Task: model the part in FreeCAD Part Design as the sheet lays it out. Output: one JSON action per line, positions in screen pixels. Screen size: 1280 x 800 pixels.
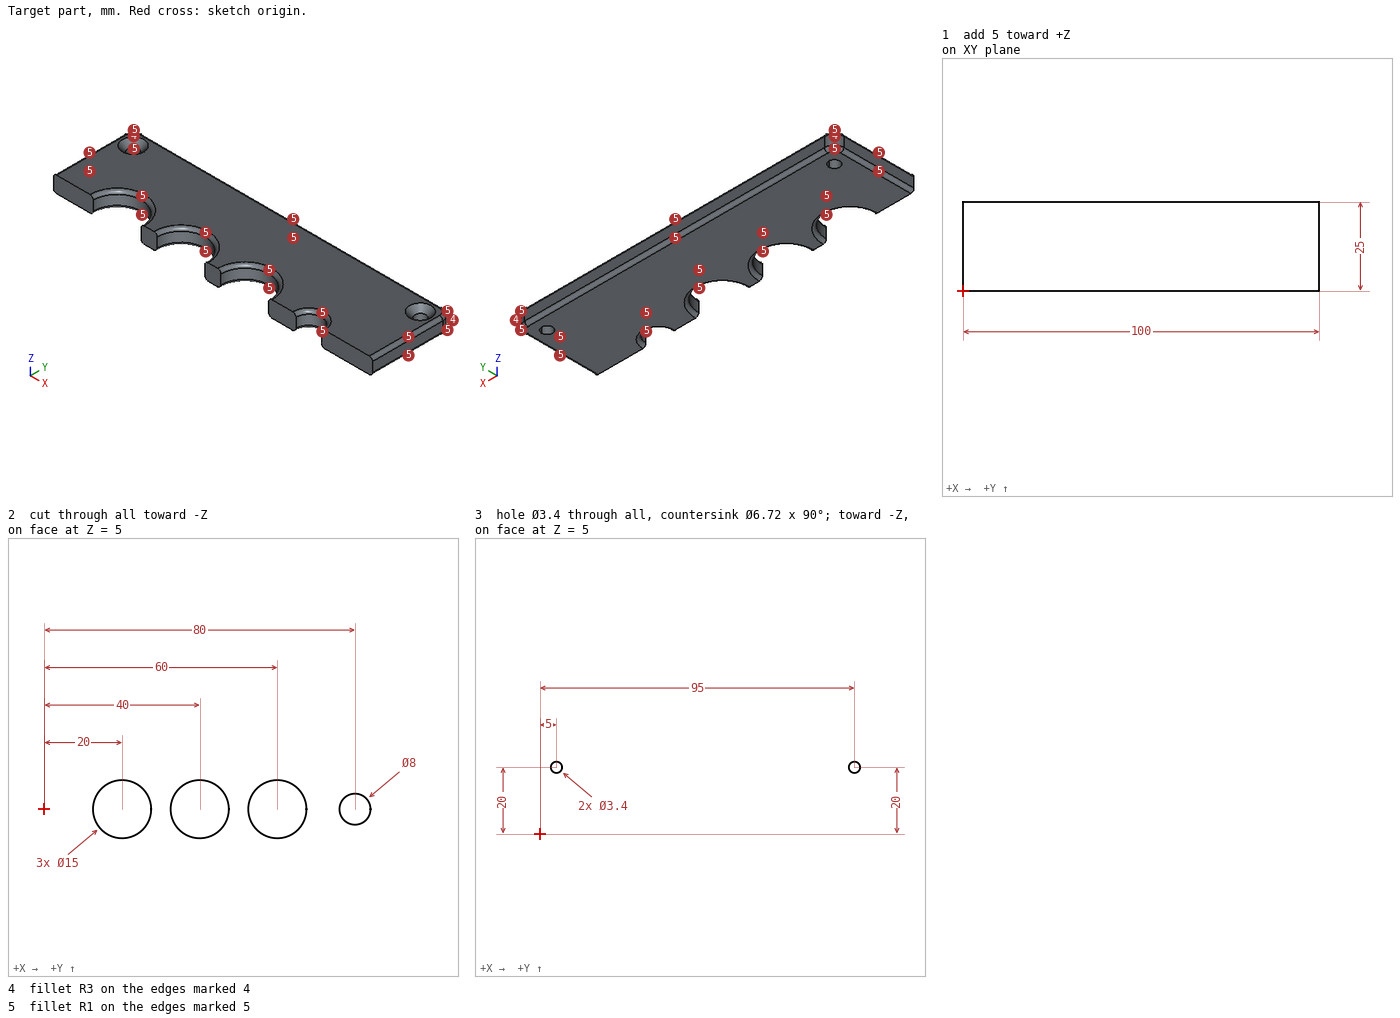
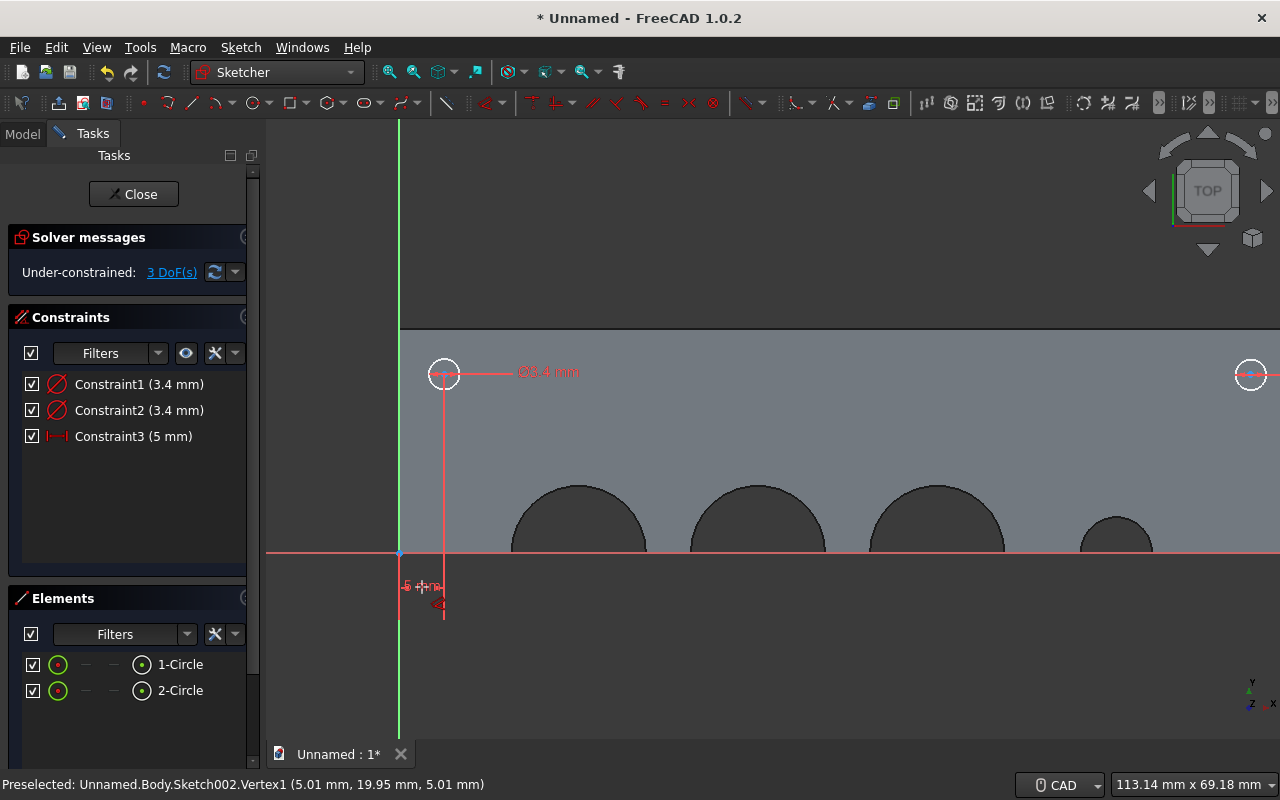
{"action": "left_click", "coordinate": [444, 374]}
{"action": "left_click", "coordinate": [365, 464]}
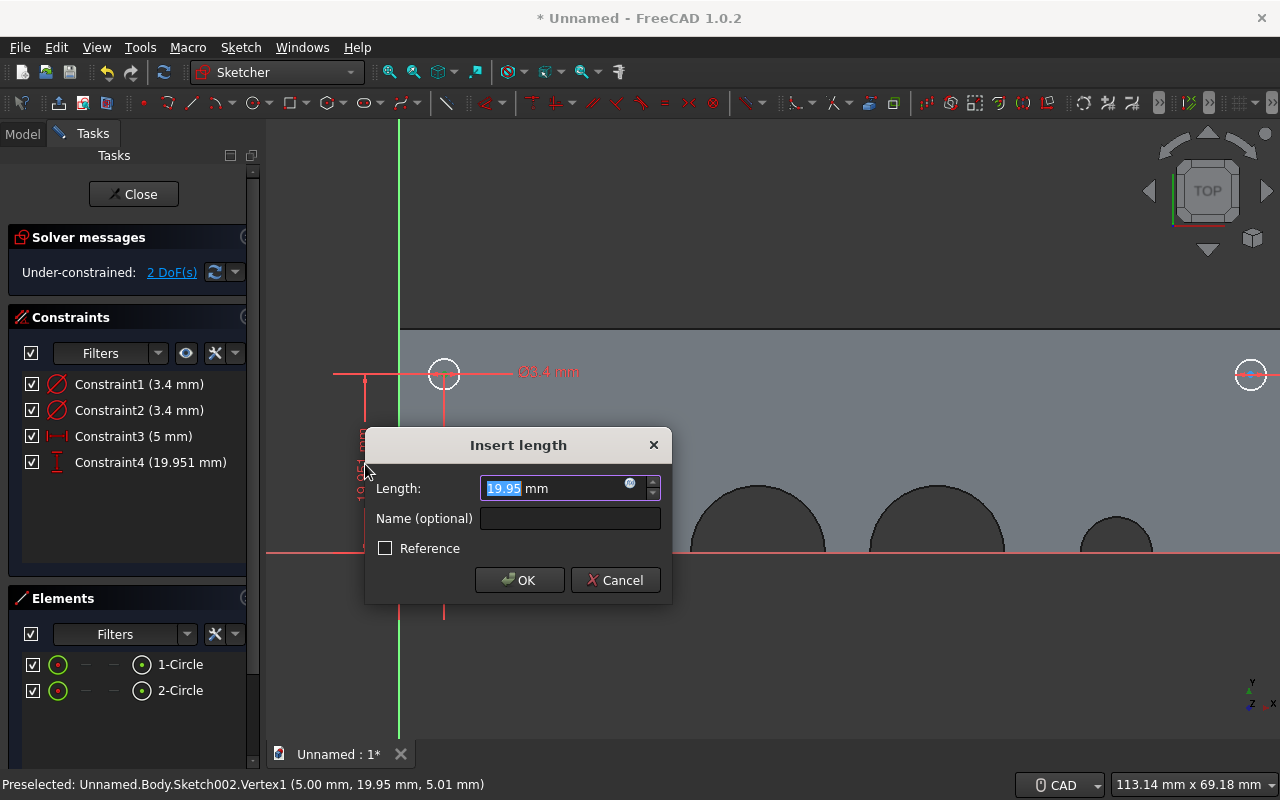
{"action": "type", "text": "20"}
{"action": "key", "text": "Return"}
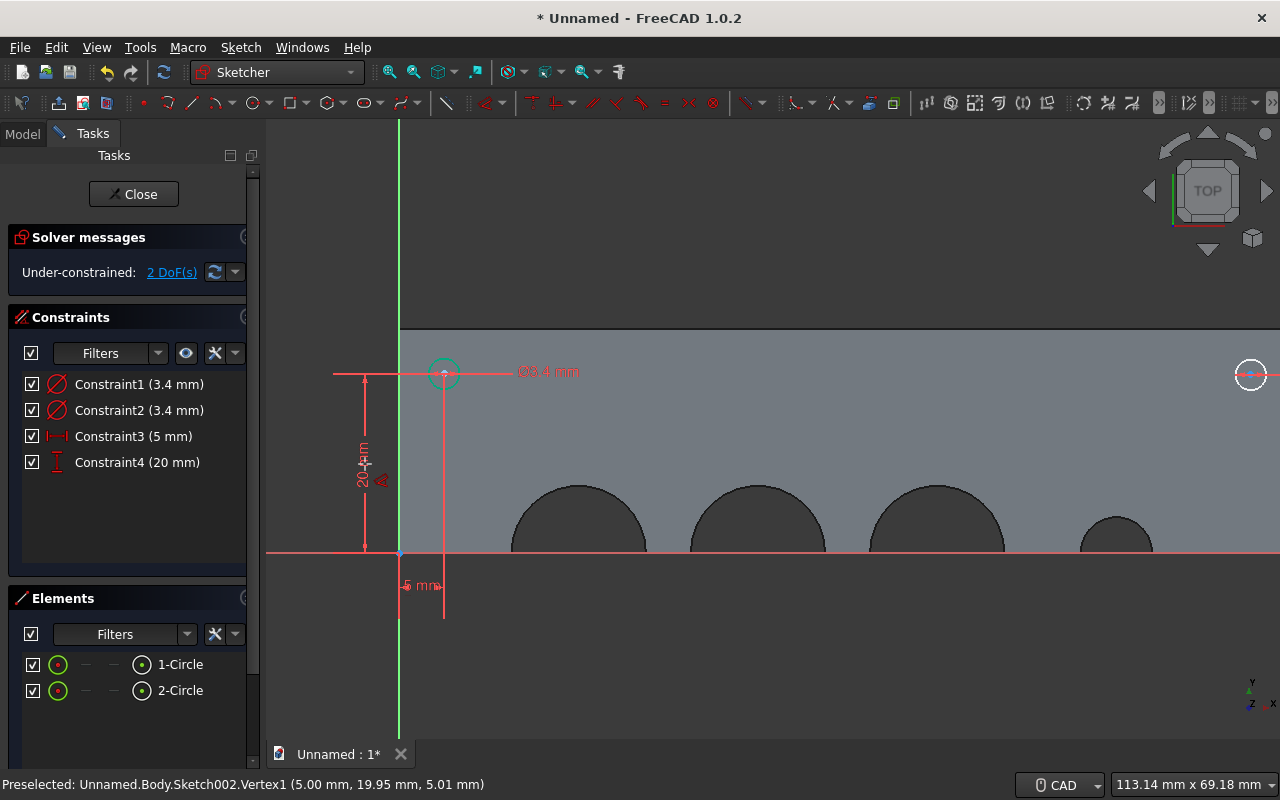
{"action": "scroll", "coordinate": [444, 374], "scroll_direction": "down", "scroll_amount": 2}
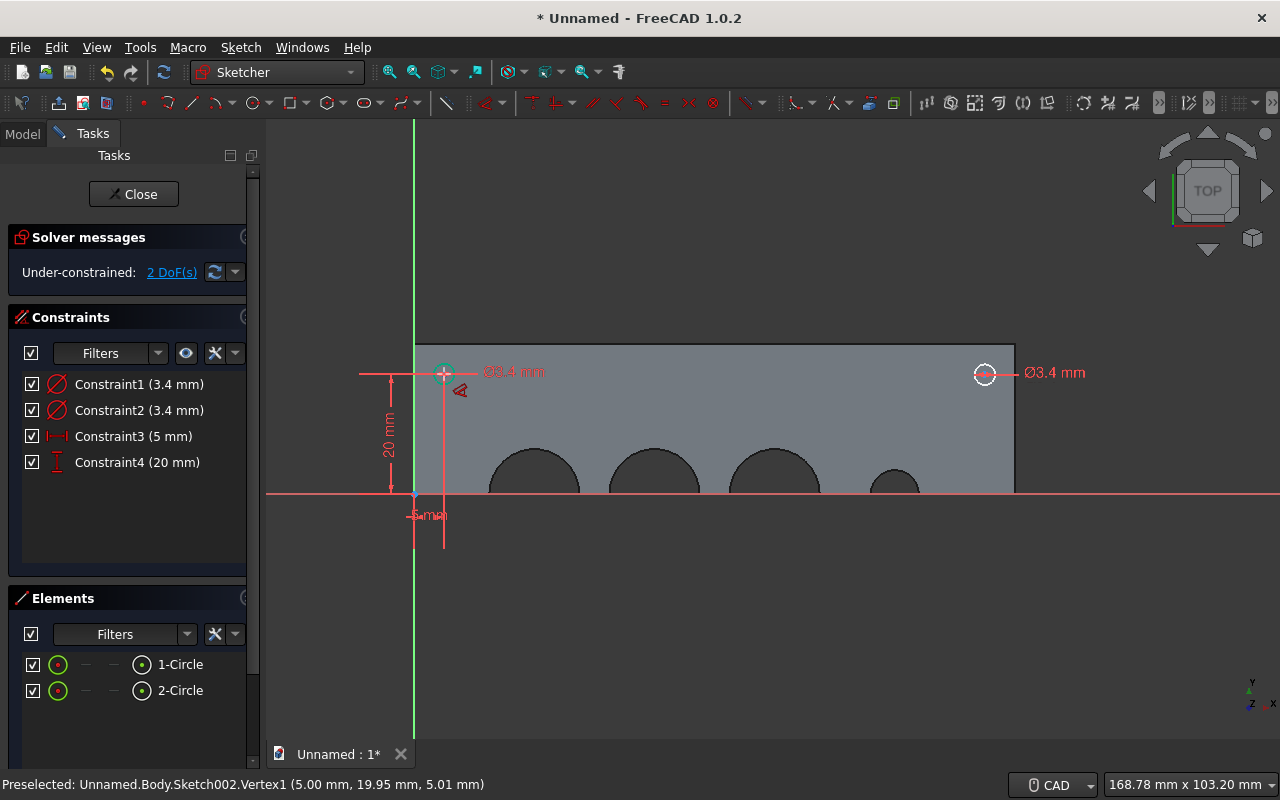
{"action": "left_click", "coordinate": [985, 375]}
{"action": "left_click", "coordinate": [700, 528]}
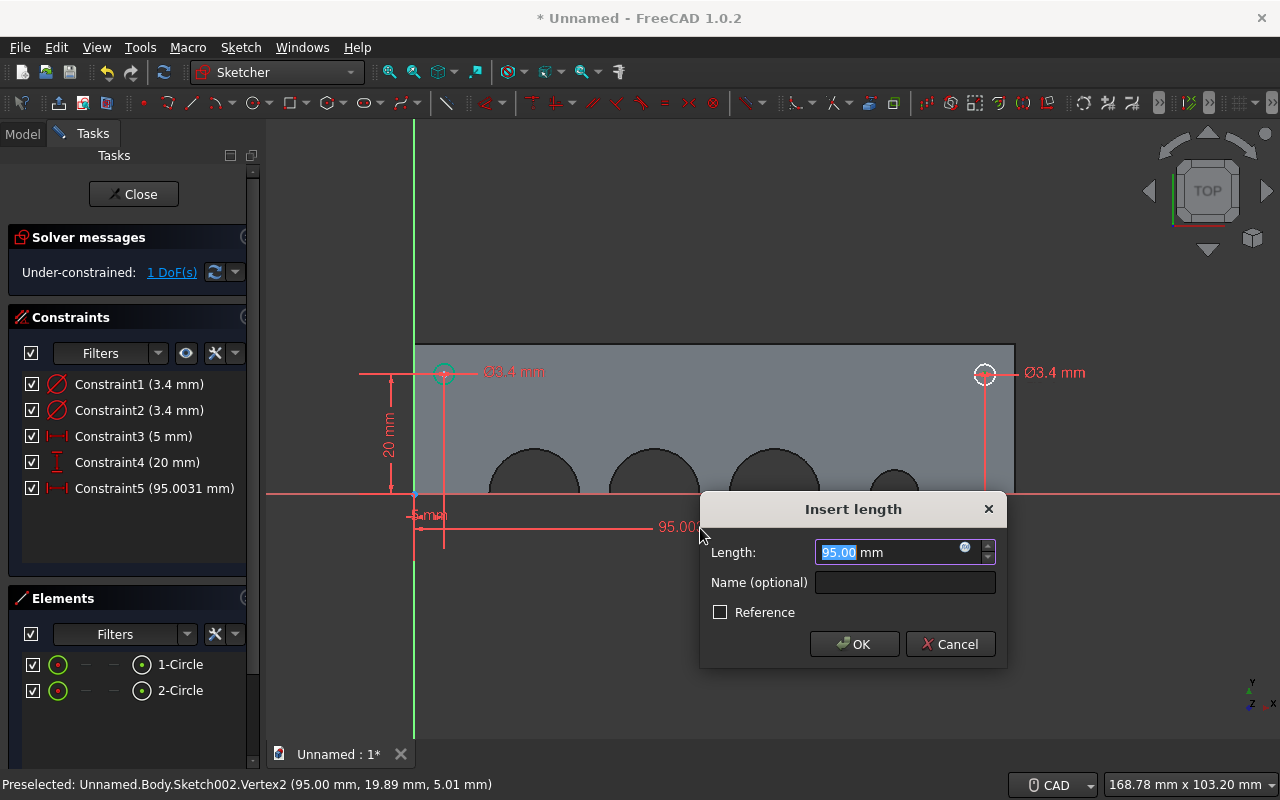
{"action": "type", "text": "95"}
{"action": "key", "text": "Return"}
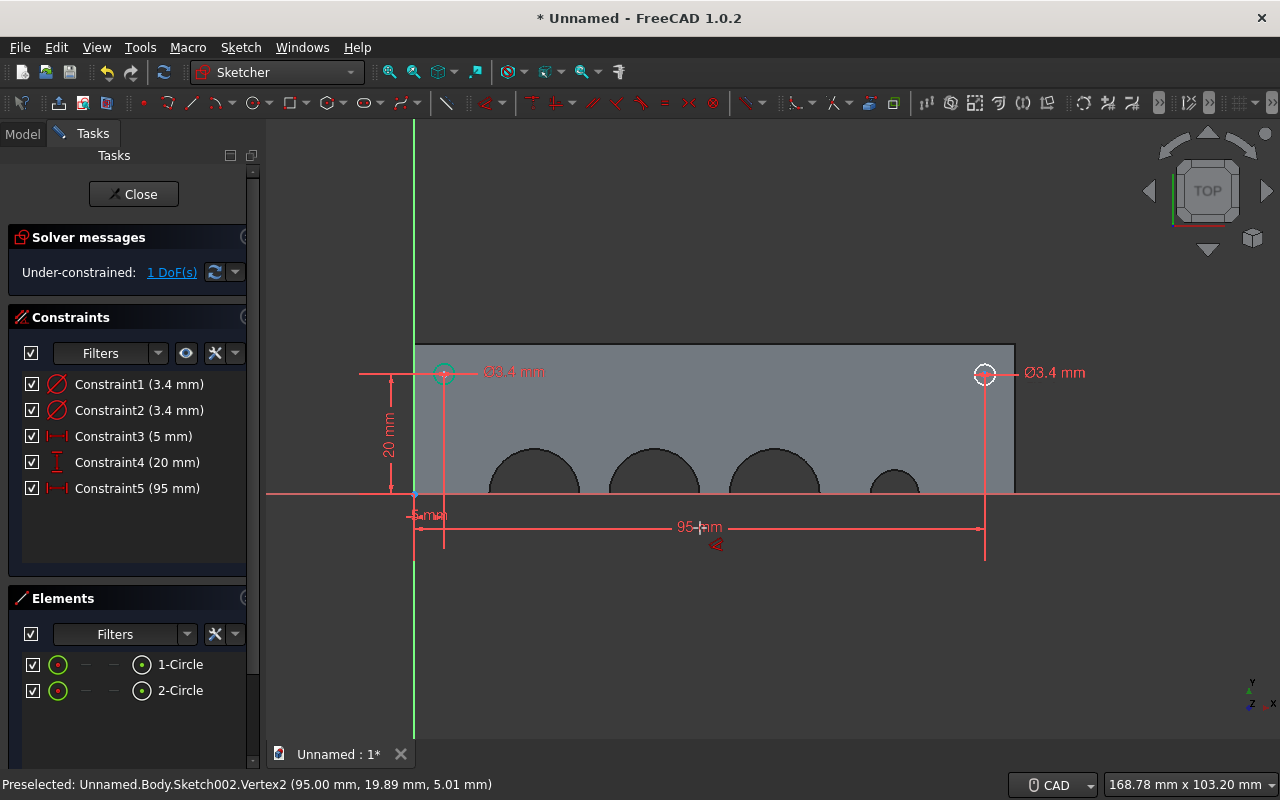
{"action": "left_click", "coordinate": [985, 375]}
{"action": "left_click", "coordinate": [380, 407]}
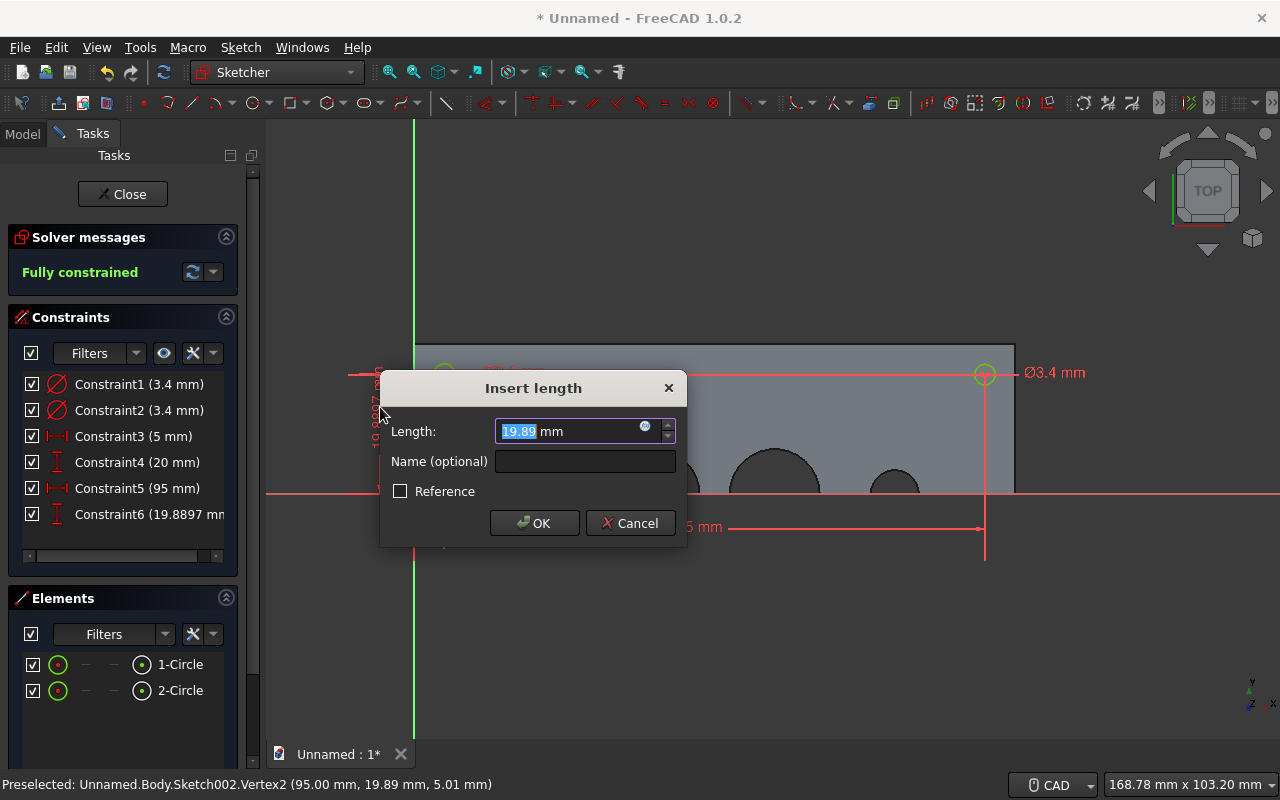
{"action": "type", "text": "20"}
{"action": "key", "text": "Return"}
{"action": "key", "text": "Escape"}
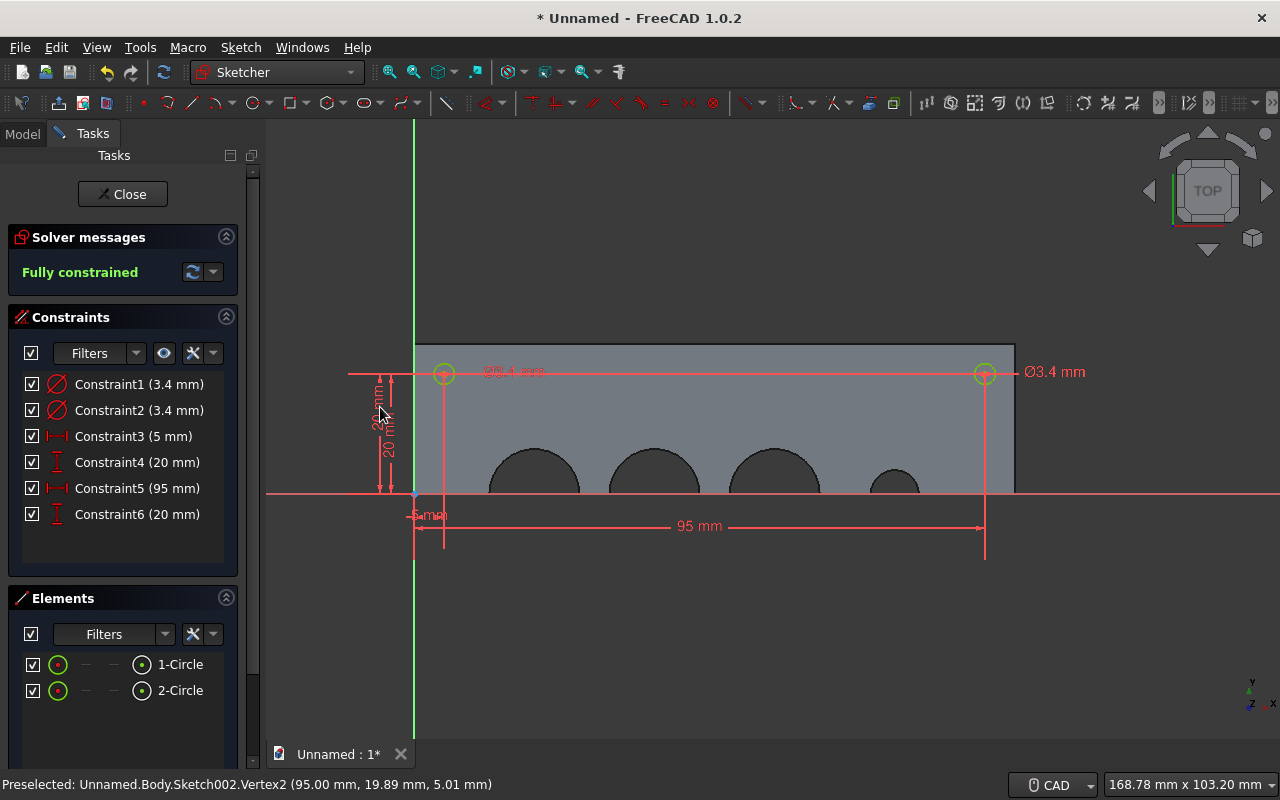
{"action": "left_click", "coordinate": [123, 194]}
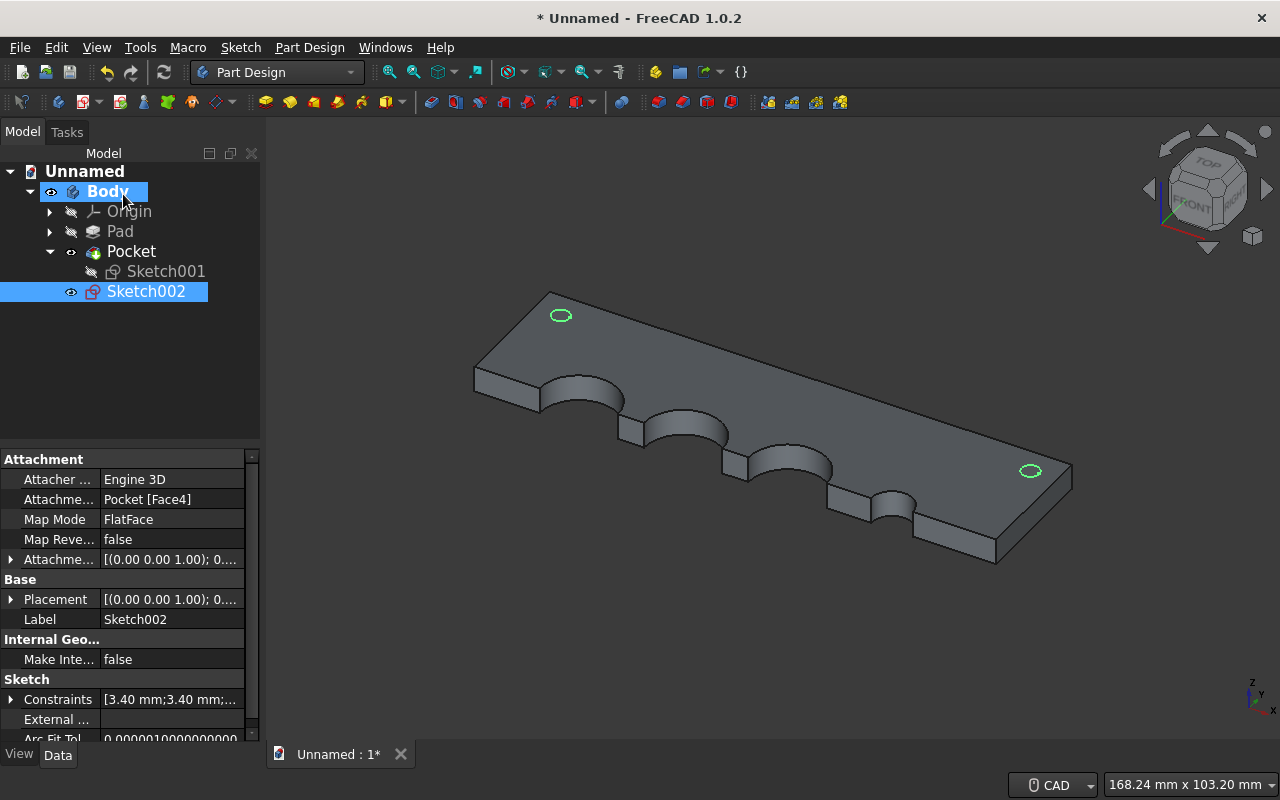
{"action": "left_click", "coordinate": [456, 102]}